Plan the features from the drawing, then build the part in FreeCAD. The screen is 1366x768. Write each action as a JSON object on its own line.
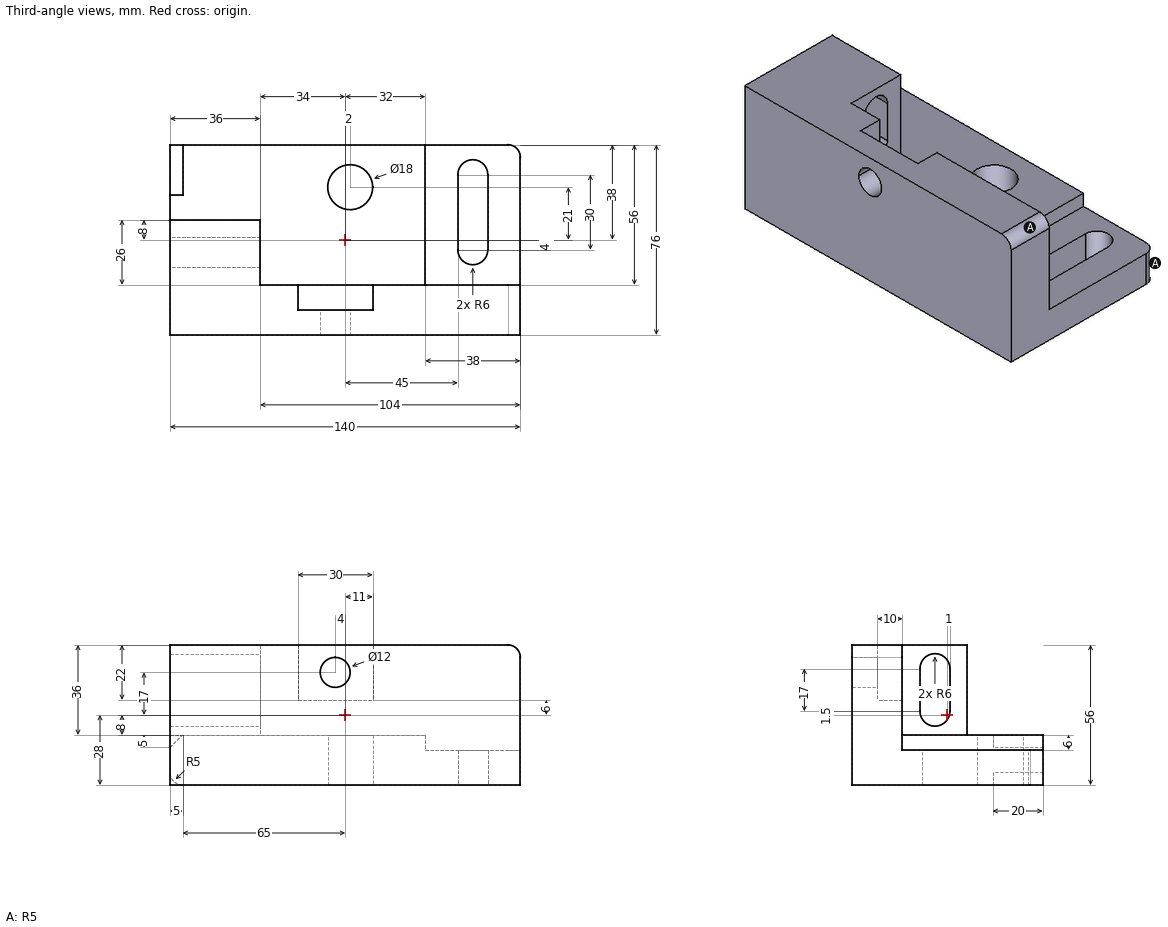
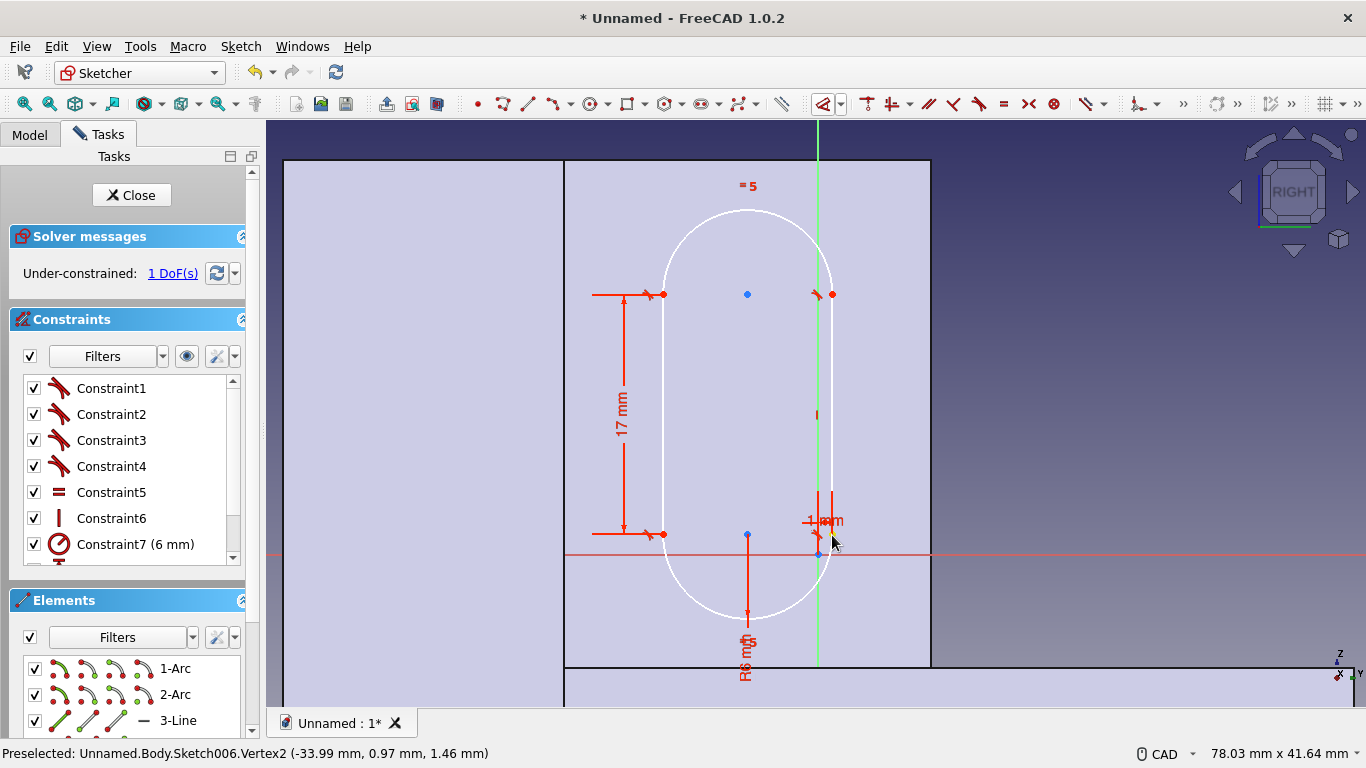
{"action": "scroll", "coordinate": [663, 534], "scroll_direction": "up", "scroll_amount": 4}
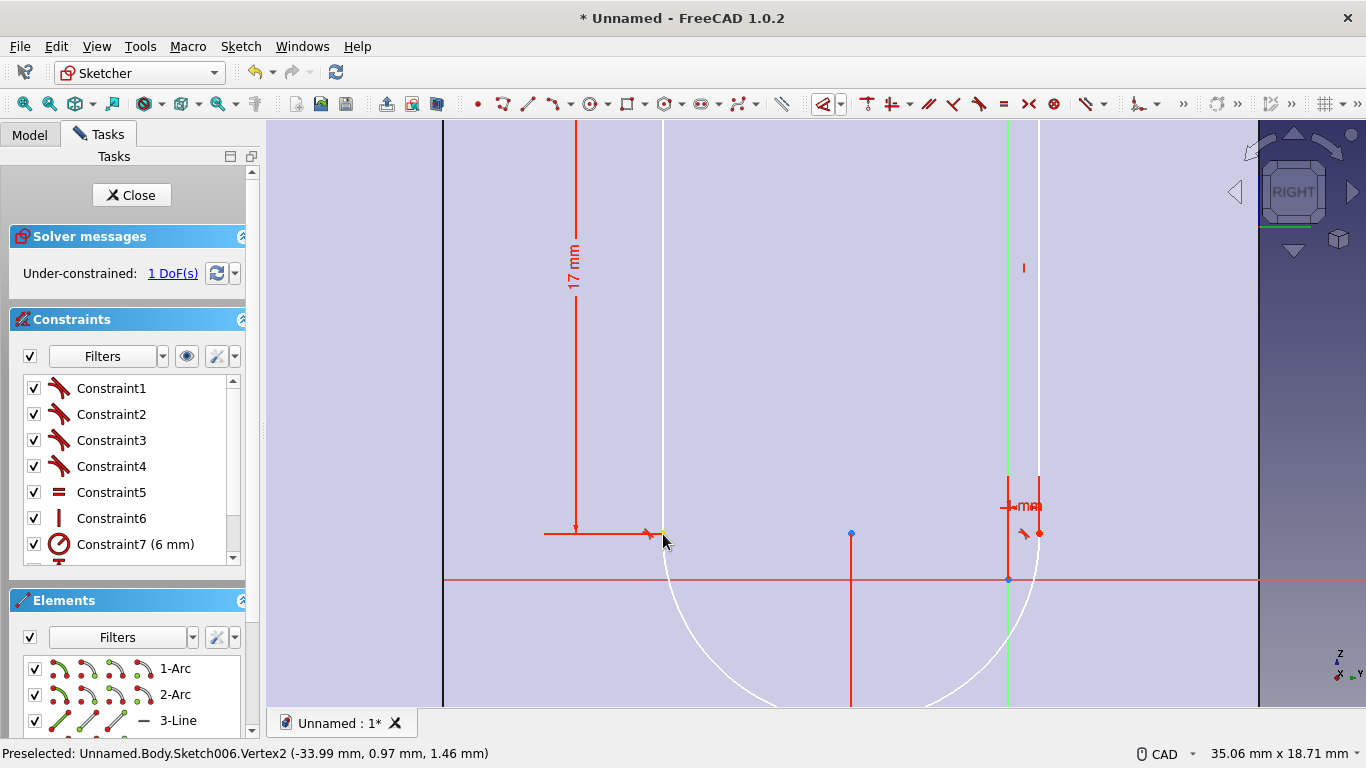
{"action": "left_click", "coordinate": [663, 534]}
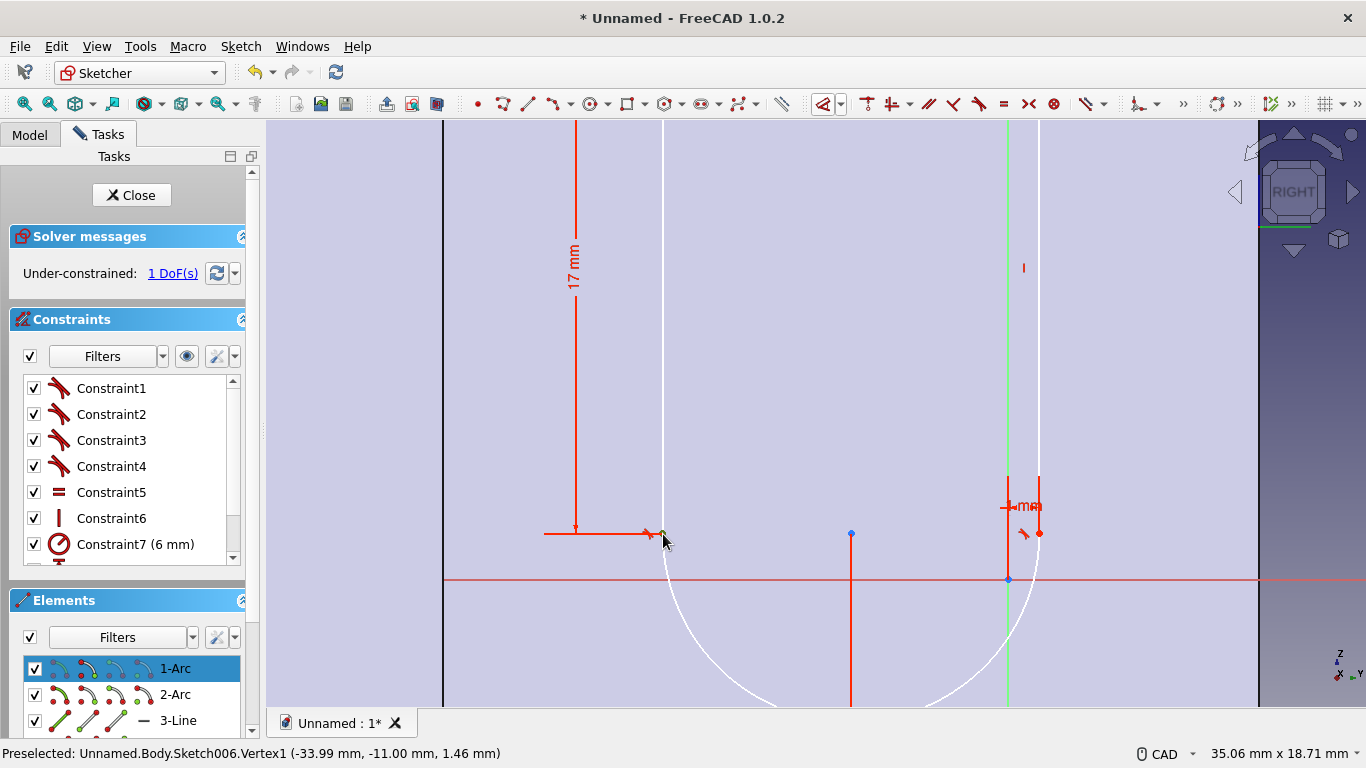
{"action": "key", "text": "i"}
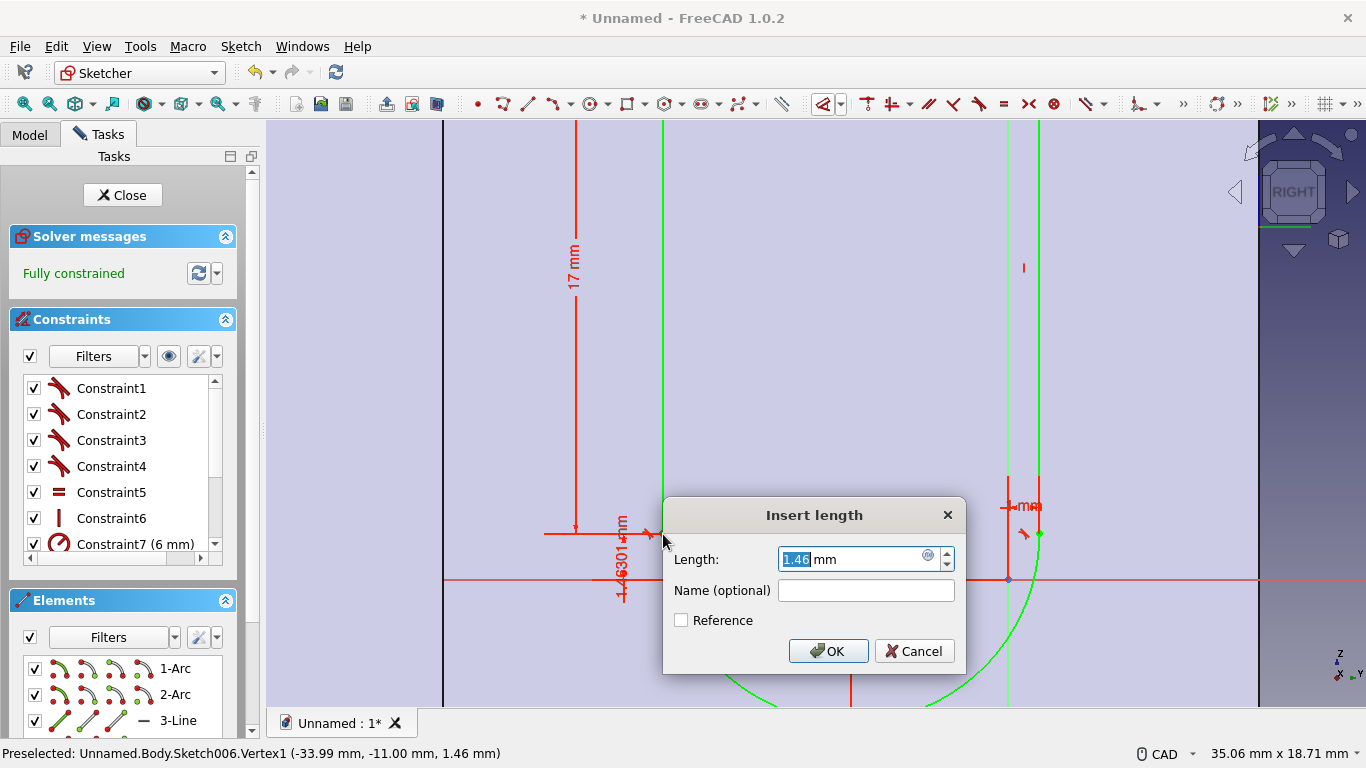
{"action": "type", "text": "1.5"}
{"action": "key", "text": "Return"}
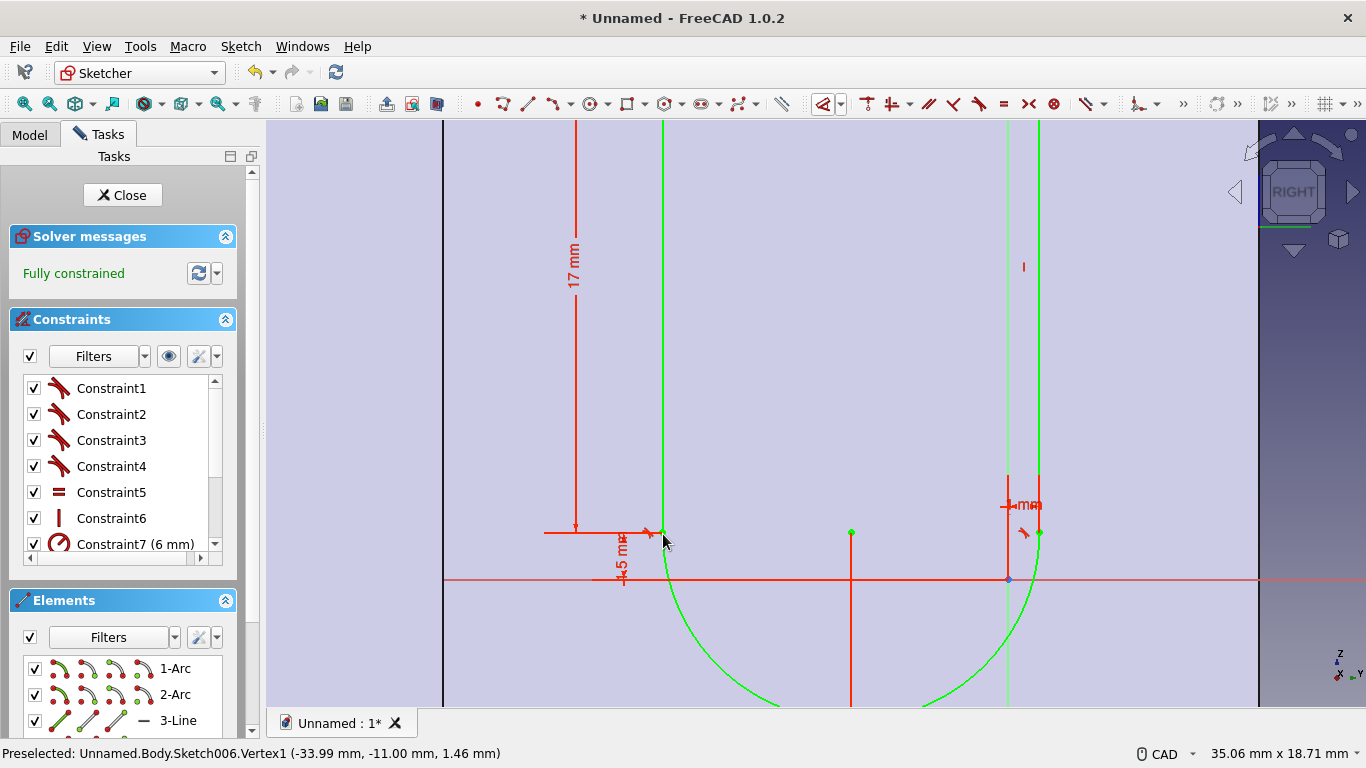
{"action": "left_click", "coordinate": [123, 195]}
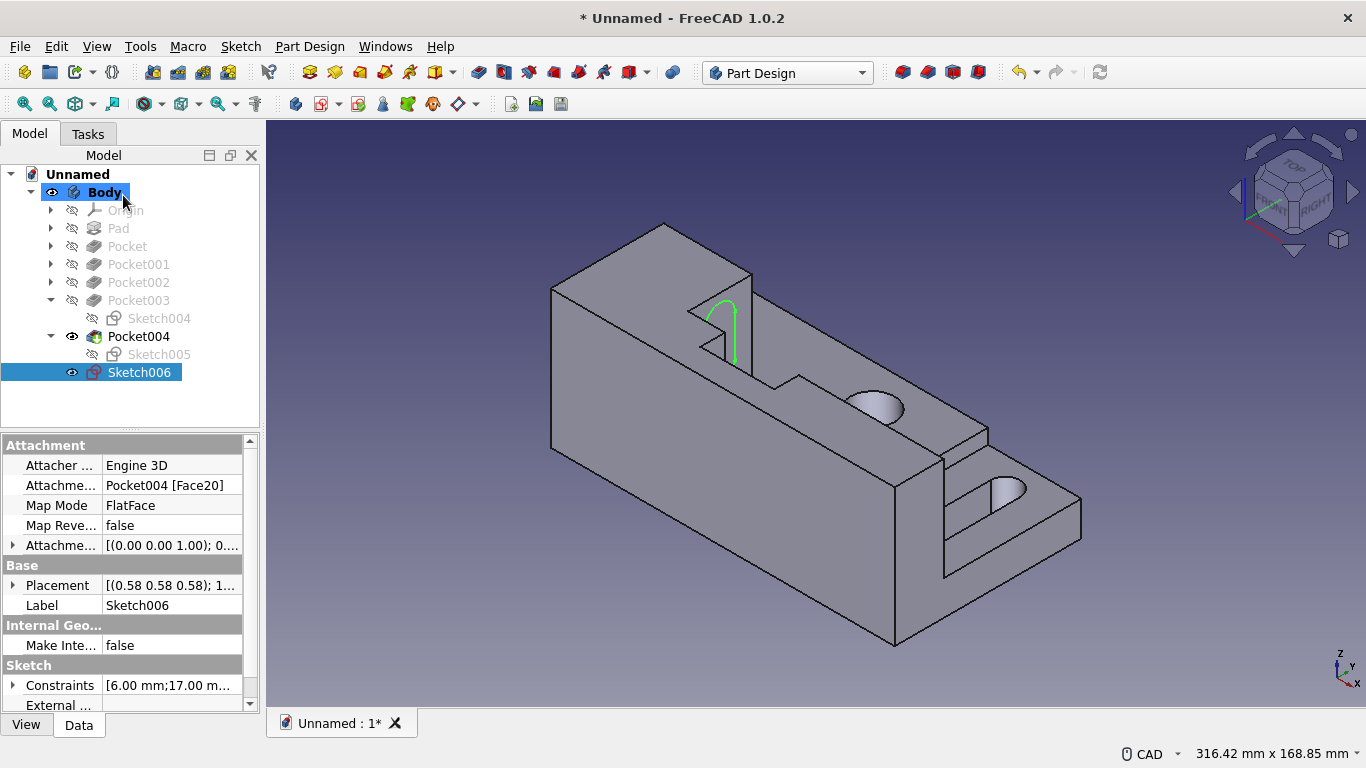
{"action": "left_click", "coordinate": [479, 72]}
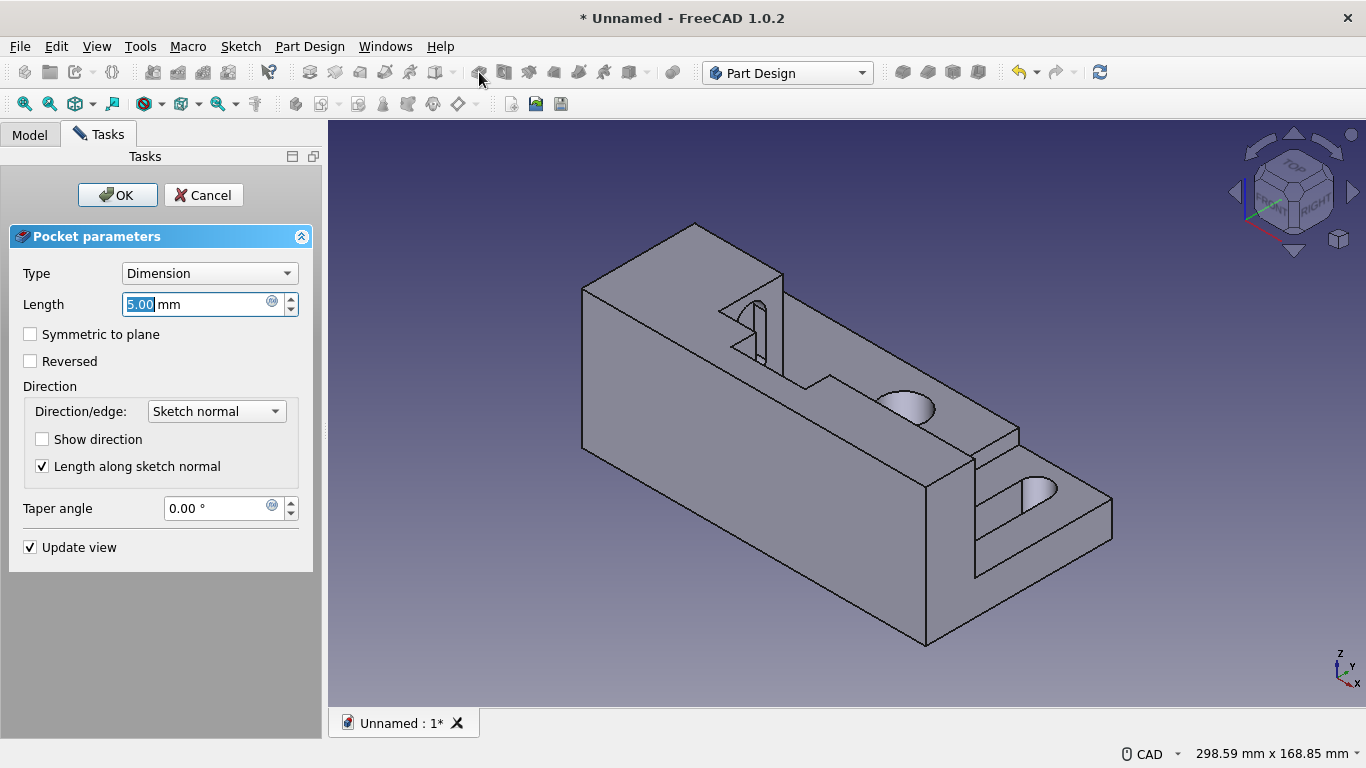
{"action": "left_click", "coordinate": [210, 274]}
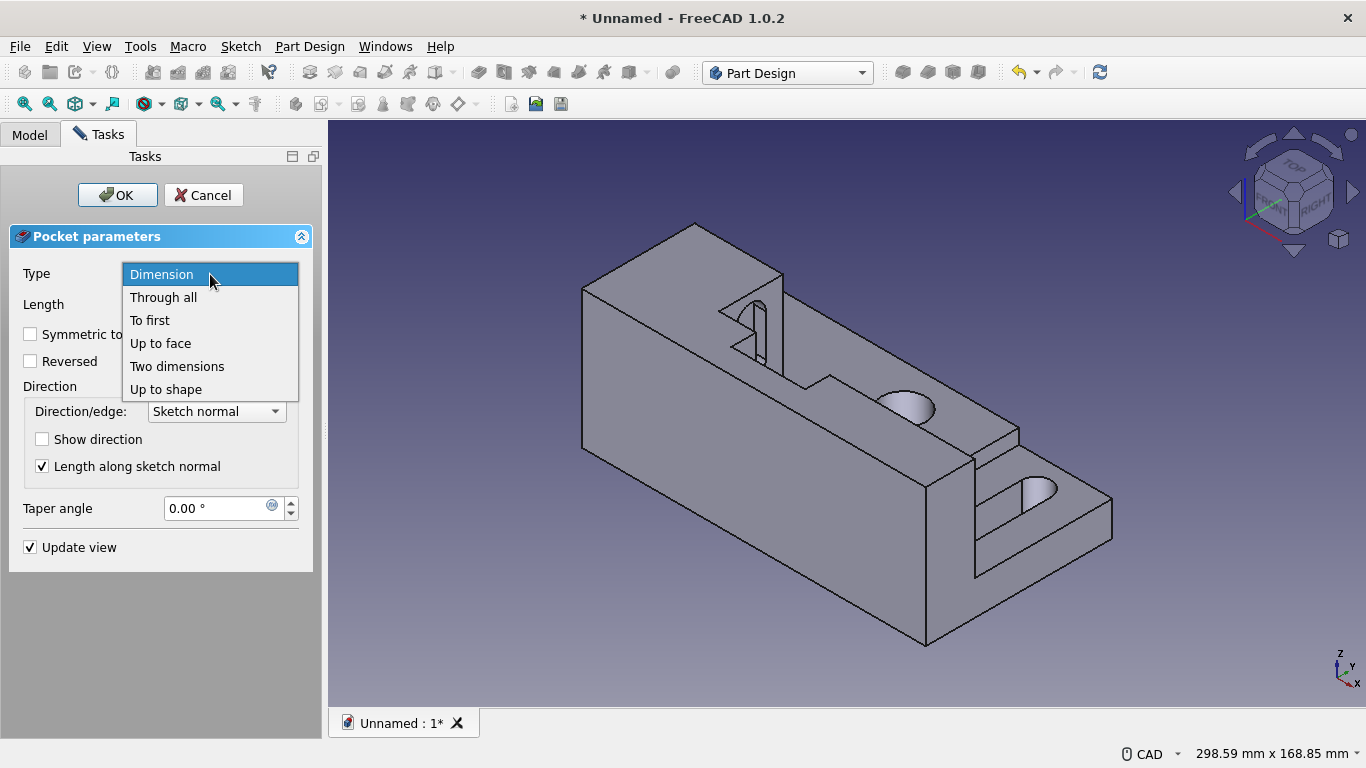
{"action": "left_click", "coordinate": [208, 298]}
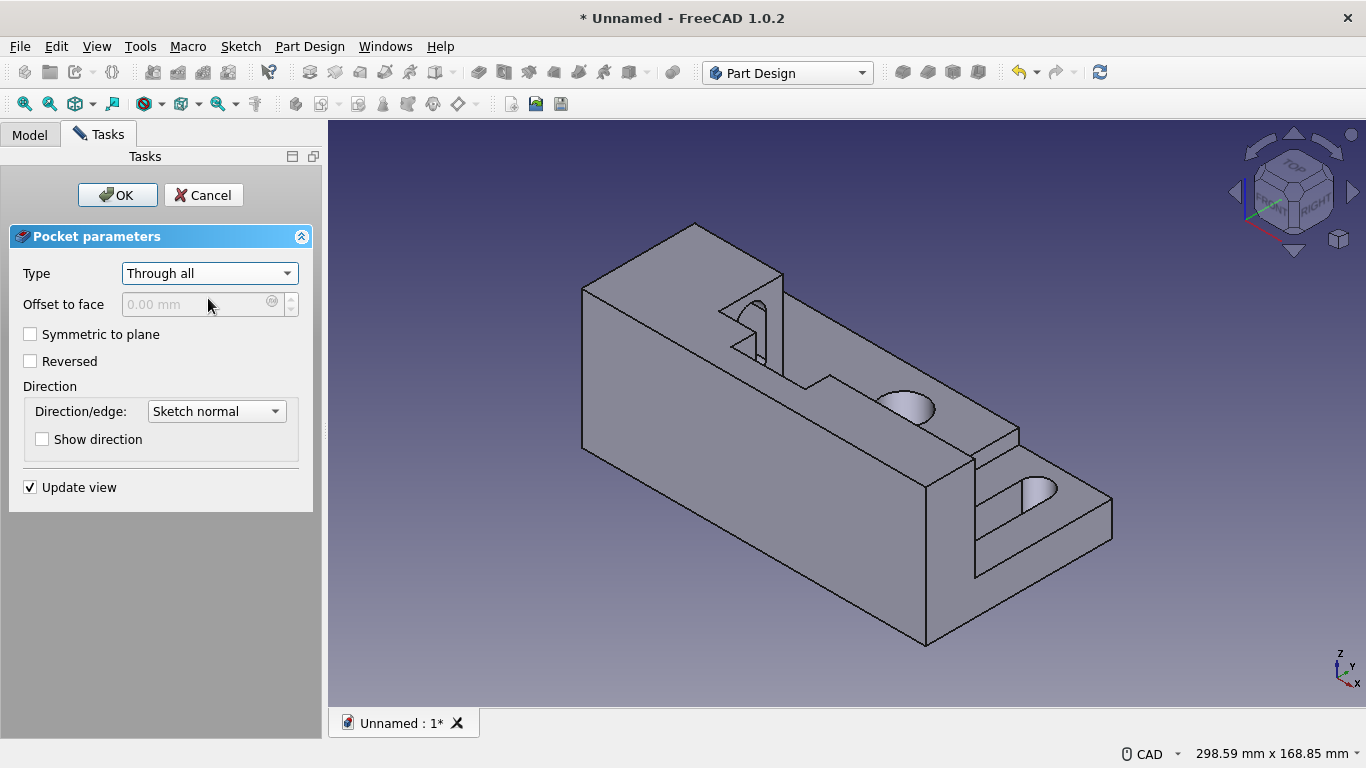
{"action": "left_click", "coordinate": [118, 195]}